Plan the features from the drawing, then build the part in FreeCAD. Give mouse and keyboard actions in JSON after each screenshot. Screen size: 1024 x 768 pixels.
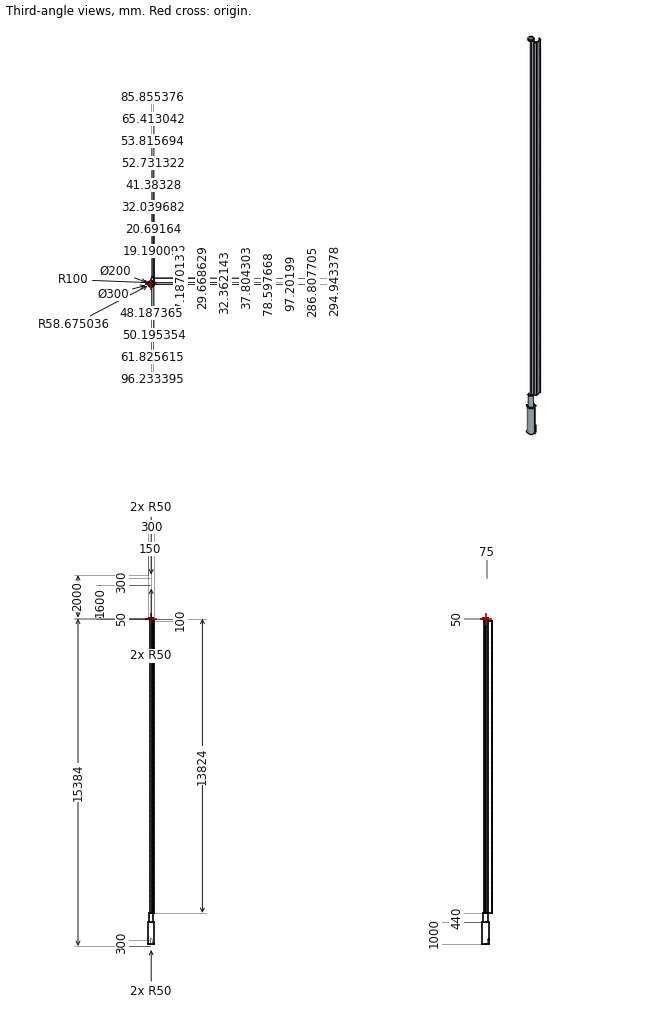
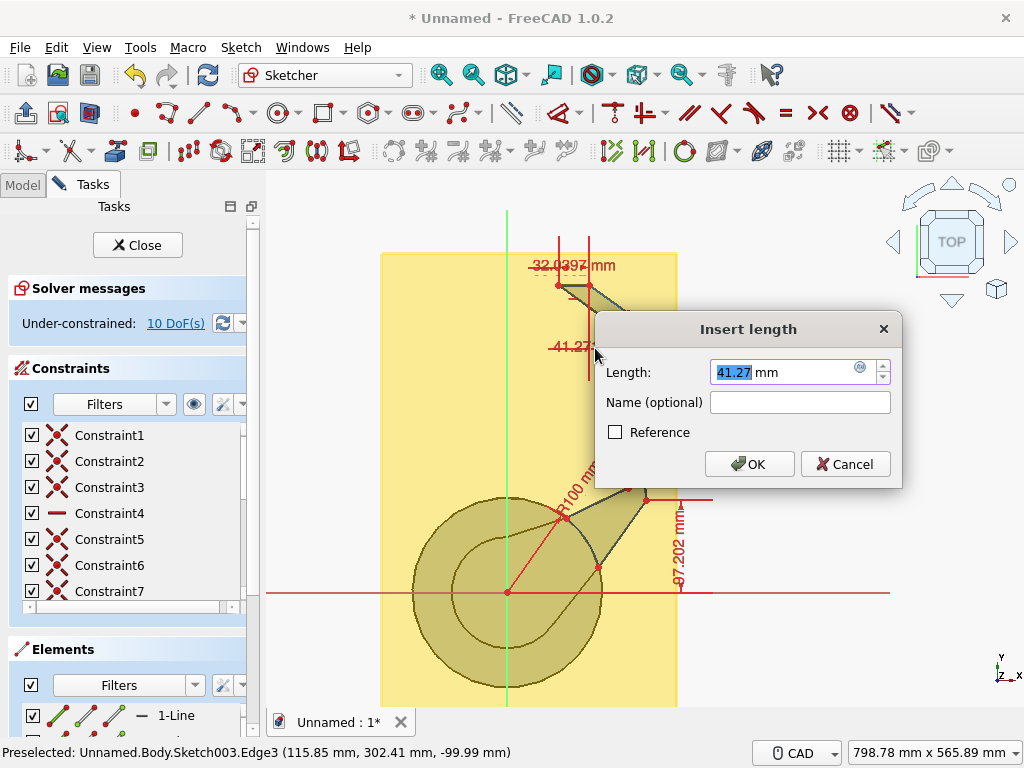
{"action": "type", "text": "41.38328"}
{"action": "key", "text": "Return"}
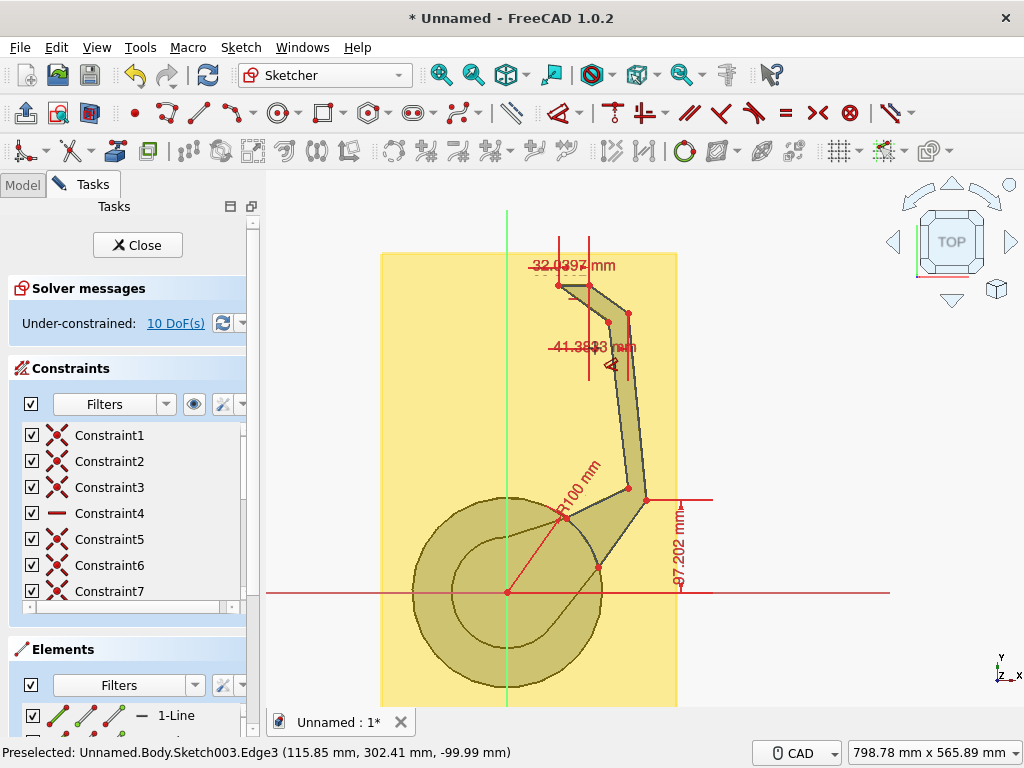
{"action": "scroll", "coordinate": [615, 372], "scroll_direction": "up", "scroll_amount": 4}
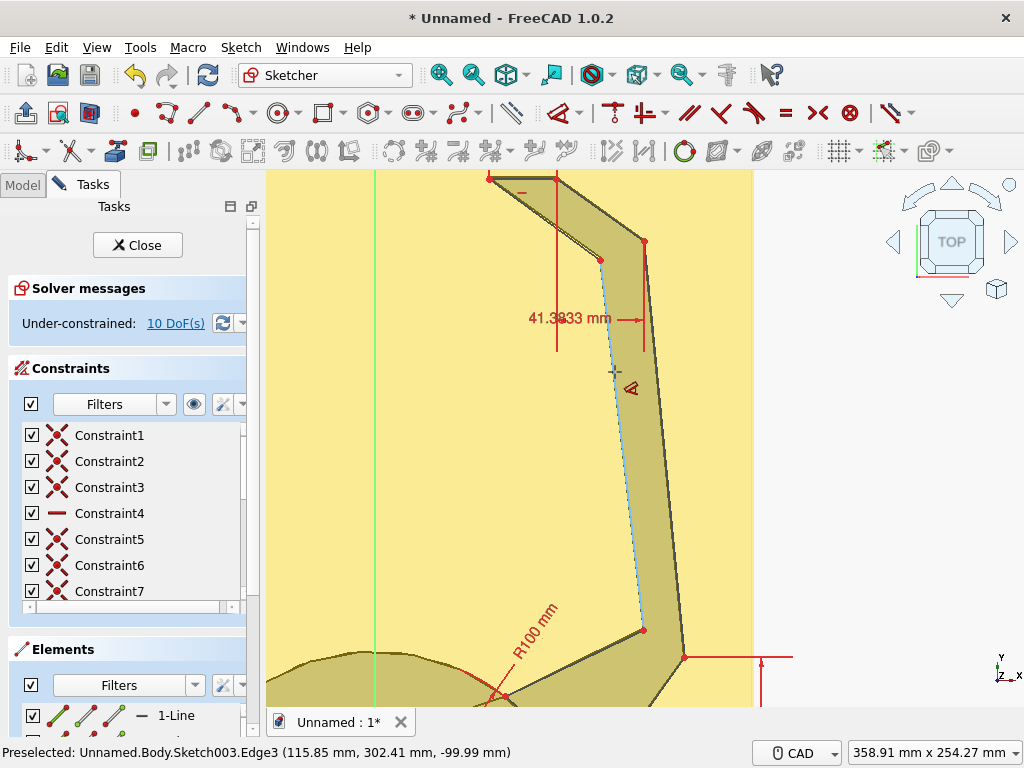
{"action": "left_click", "coordinate": [614, 371]}
{"action": "left_click", "coordinate": [622, 664]}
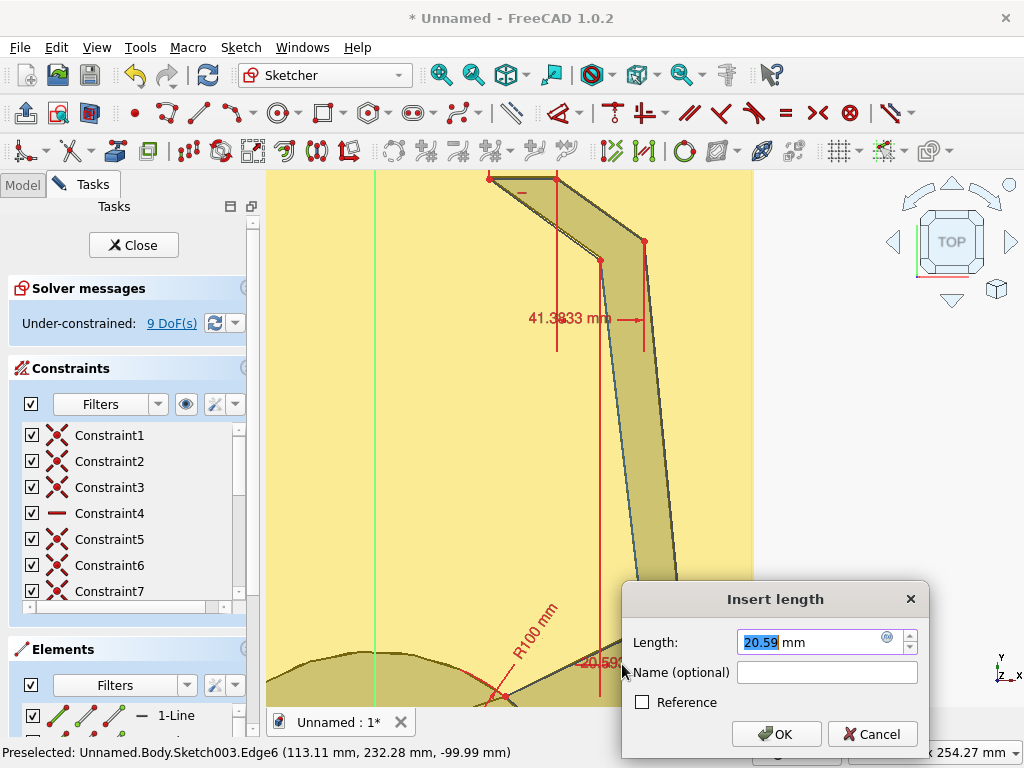
{"action": "type", "text": "20.69164"}
{"action": "key", "text": "Return"}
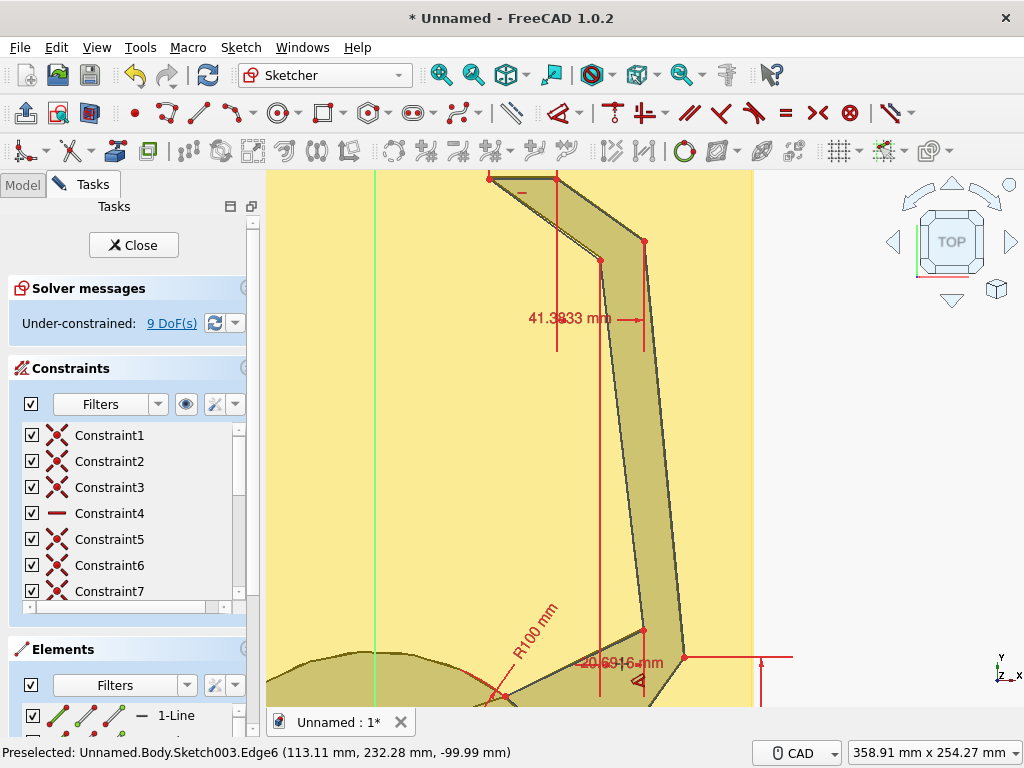
{"action": "scroll", "coordinate": [615, 372], "scroll_direction": "down", "scroll_amount": 4}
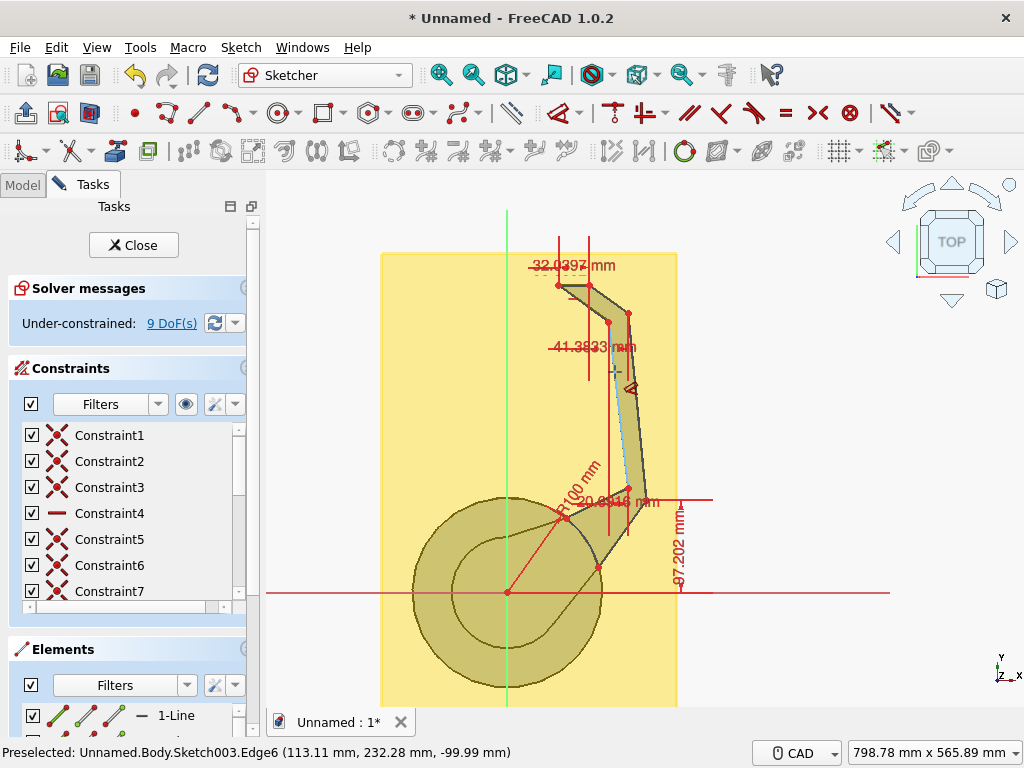
{"action": "left_click", "coordinate": [599, 568]}
{"action": "left_click", "coordinate": [553, 627]}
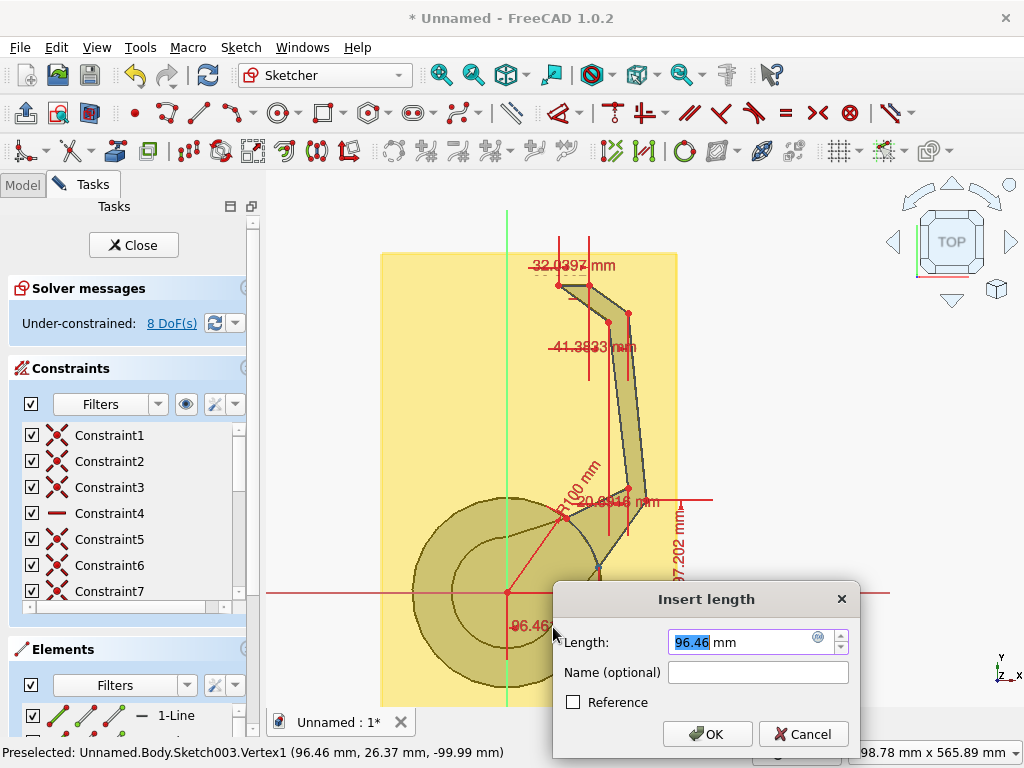
{"action": "type", "text": "96.233395"}
{"action": "key", "text": "Return"}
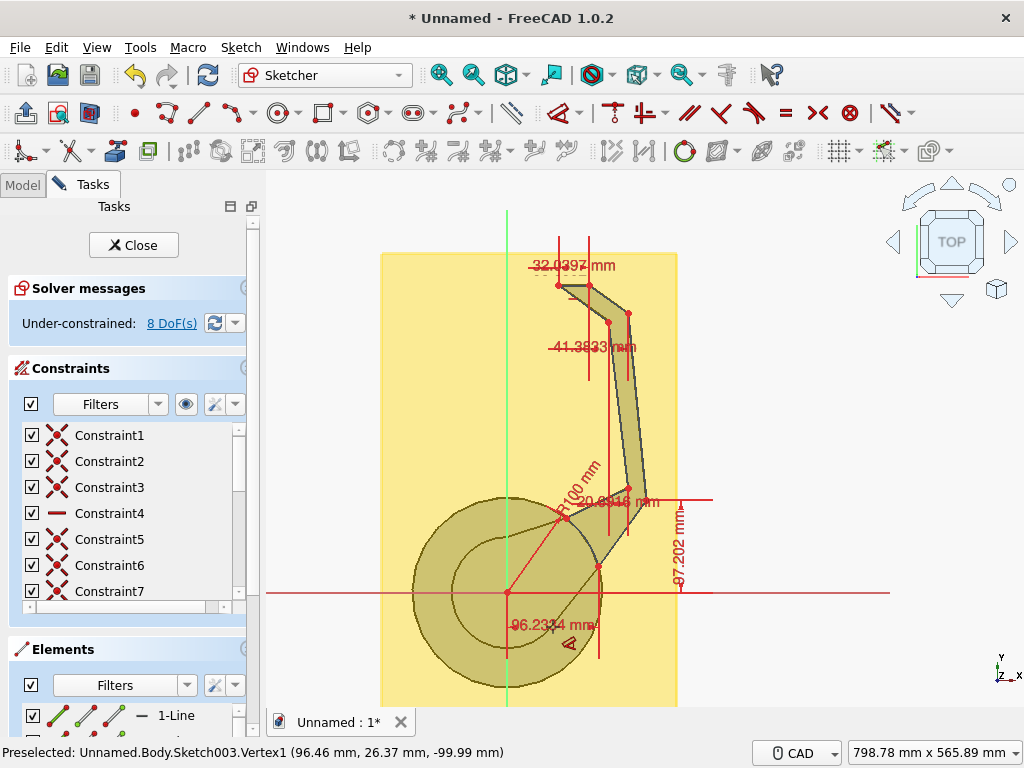
{"action": "left_click", "coordinate": [589, 286]}
{"action": "left_click", "coordinate": [548, 651]}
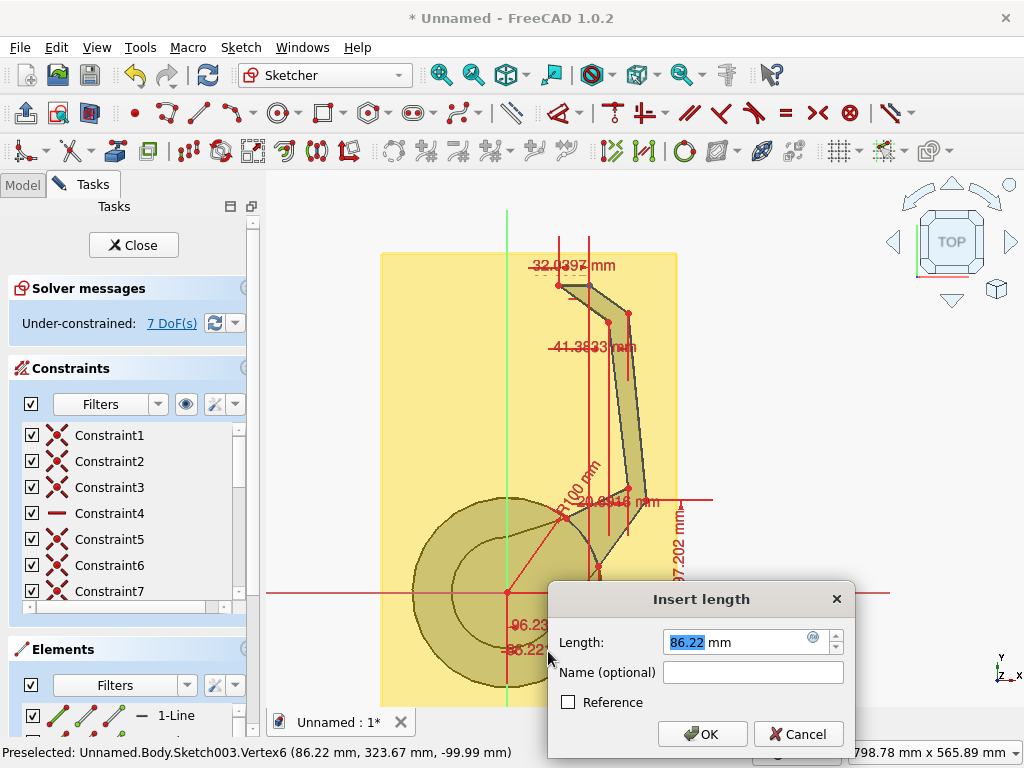
{"action": "type", "text": "85.855376"}
{"action": "key", "text": "Return"}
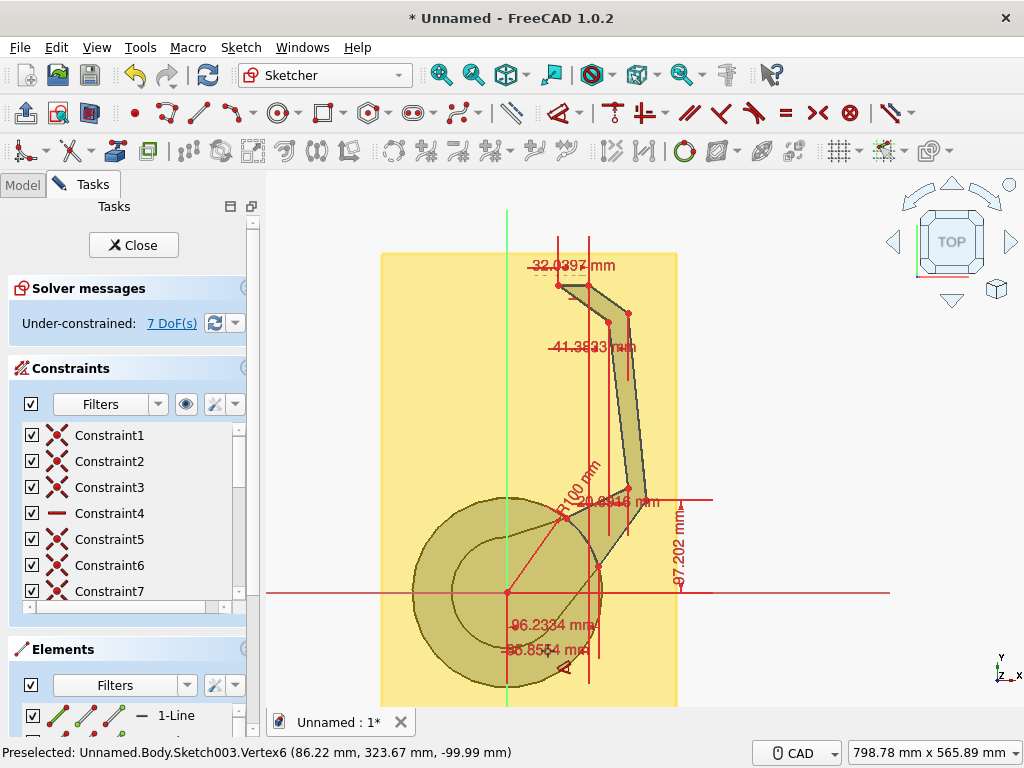
{"action": "left_click", "coordinate": [566, 518]}
{"action": "left_click", "coordinate": [537, 460]}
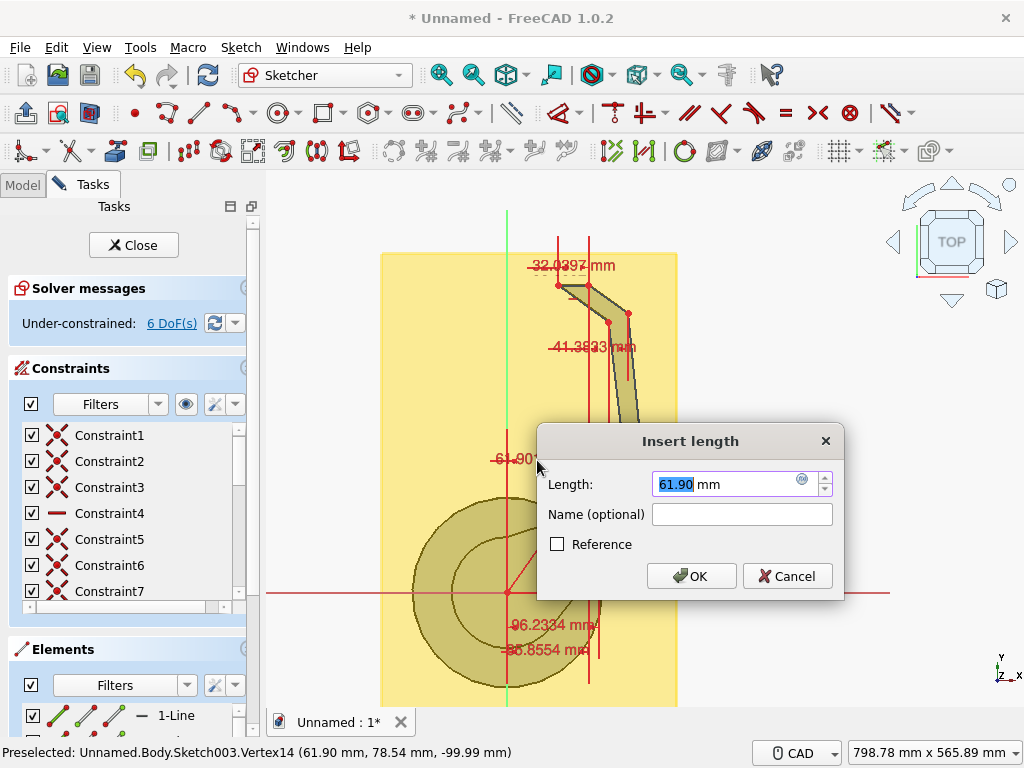
{"action": "type", "text": "61.825615"}
{"action": "key", "text": "Return"}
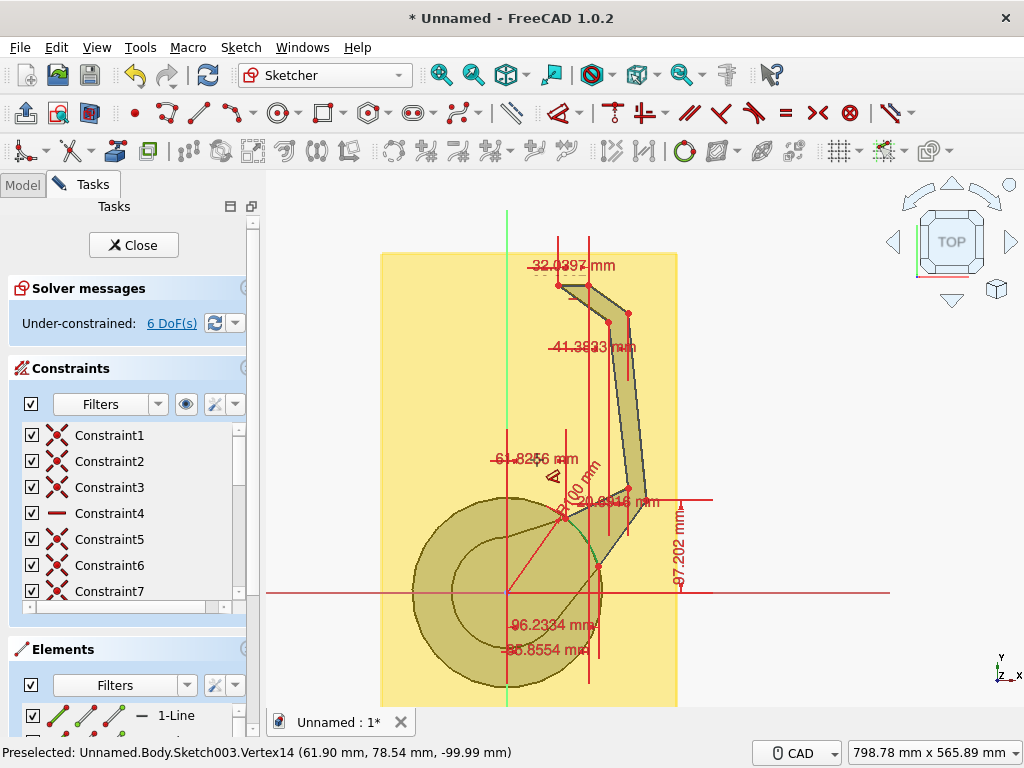
{"action": "left_click", "coordinate": [613, 547]}
{"action": "left_click", "coordinate": [612, 466]}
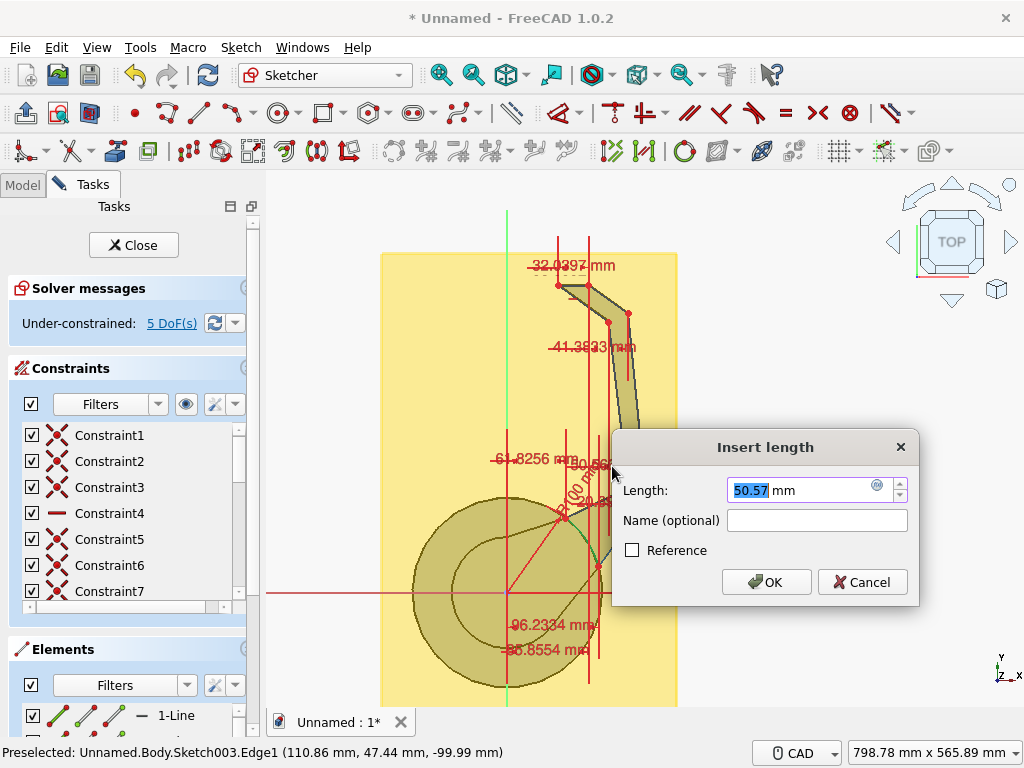
{"action": "type", "text": "50.195354"}
{"action": "key", "text": "Return"}